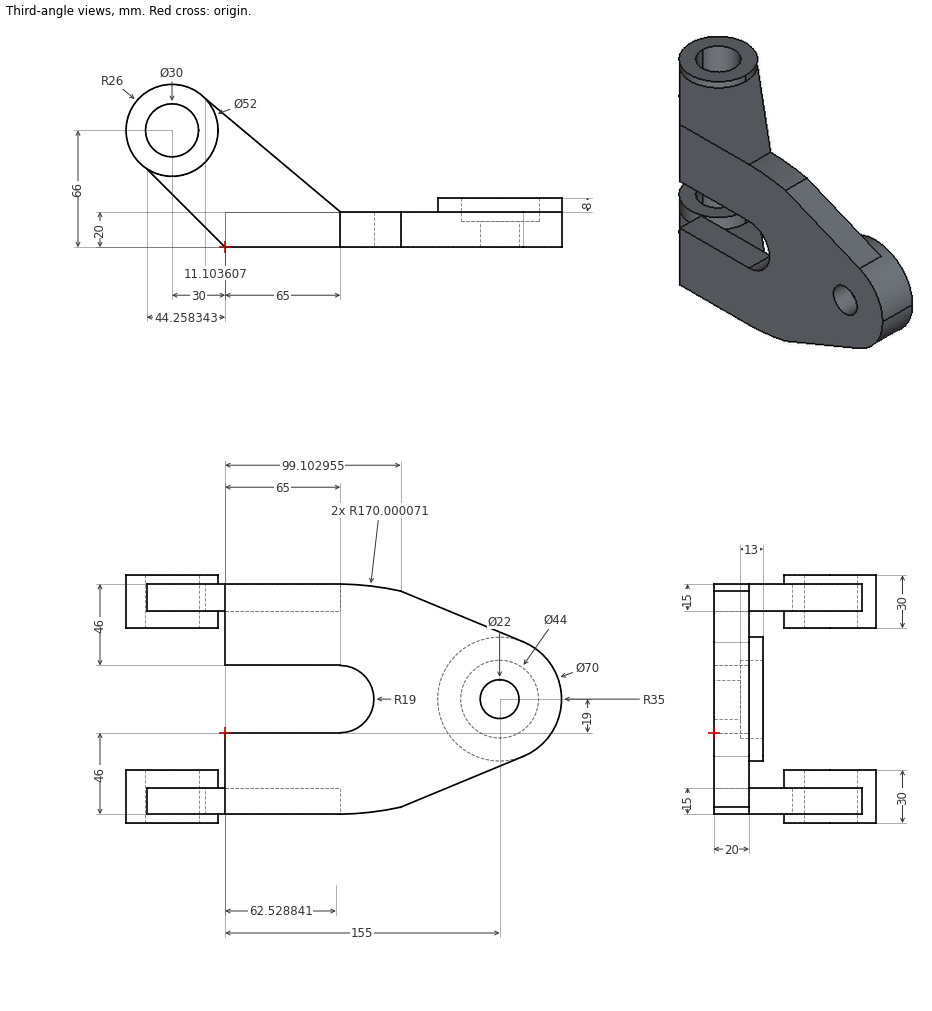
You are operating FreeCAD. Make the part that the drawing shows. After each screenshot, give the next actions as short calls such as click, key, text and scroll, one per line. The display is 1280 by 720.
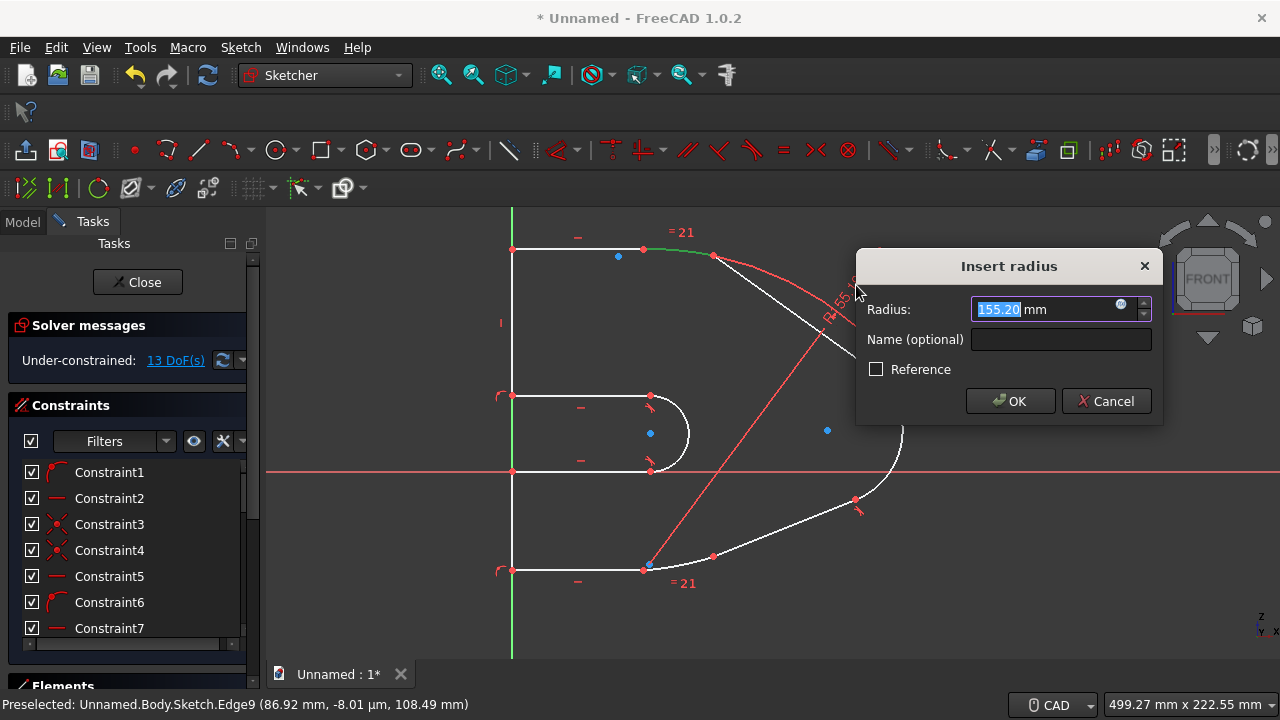
text(170.000071)
key(Return)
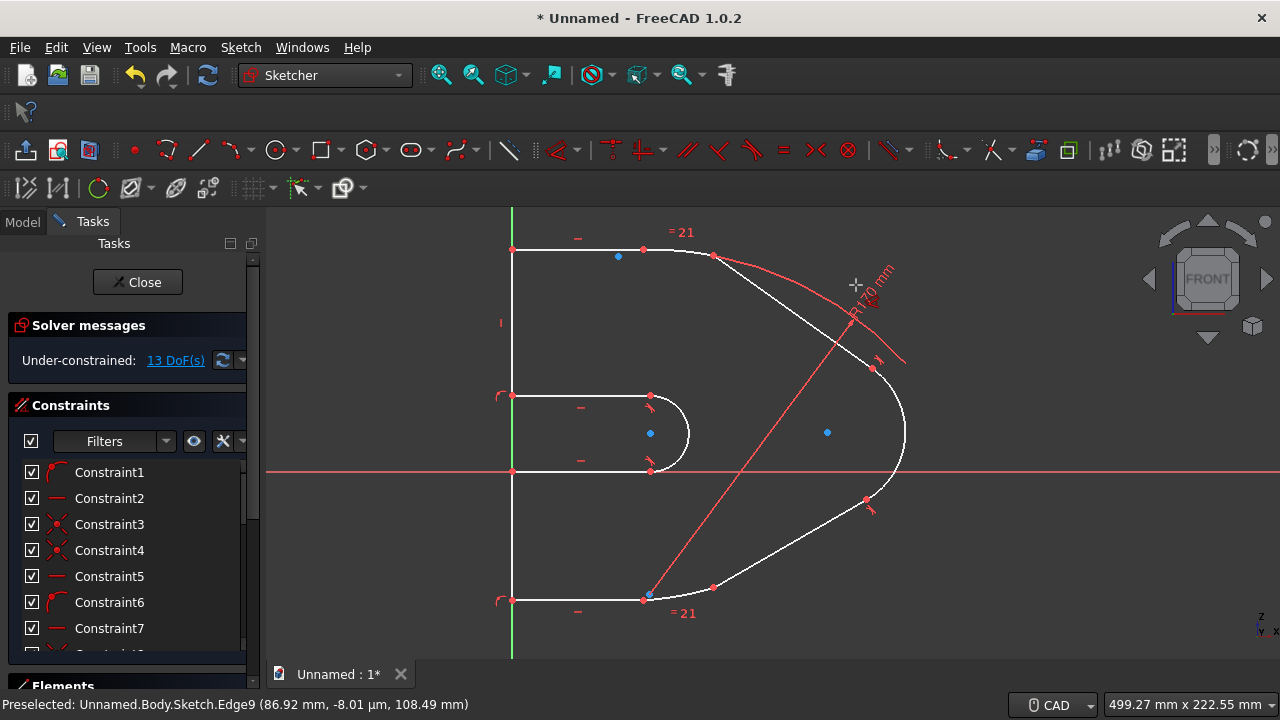
click(901, 406)
click(931, 395)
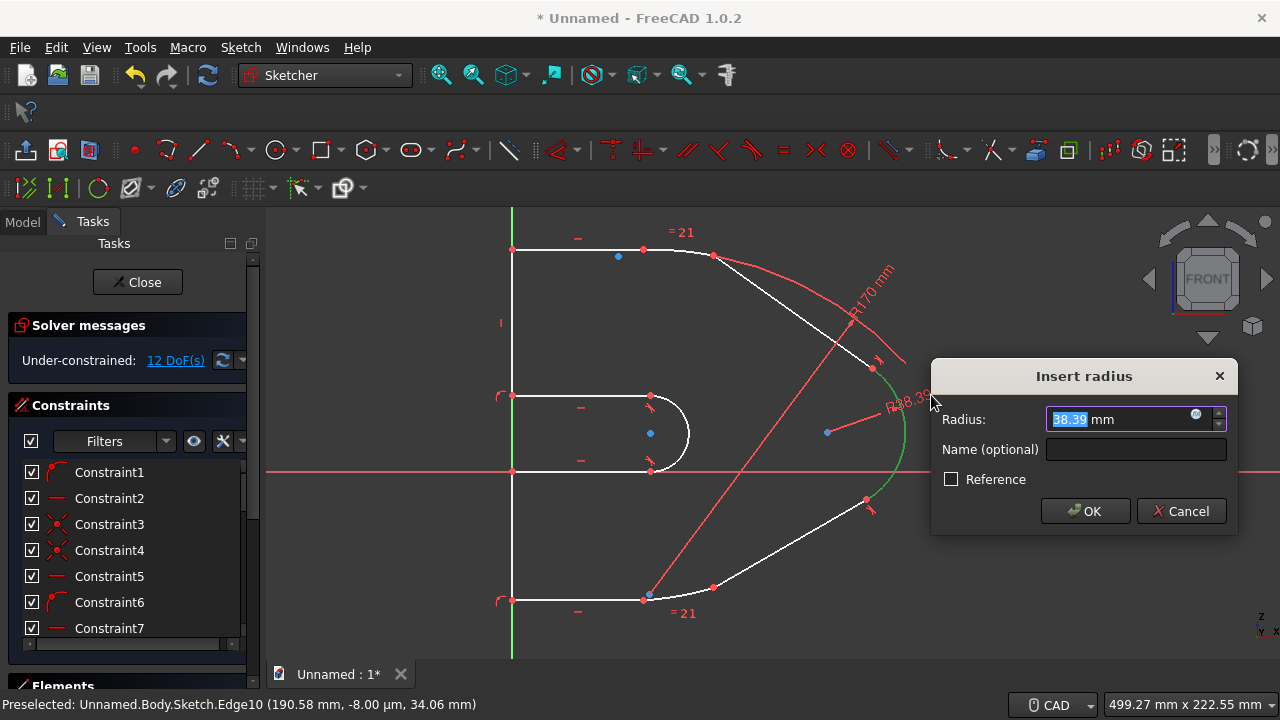
text(35)
key(Return)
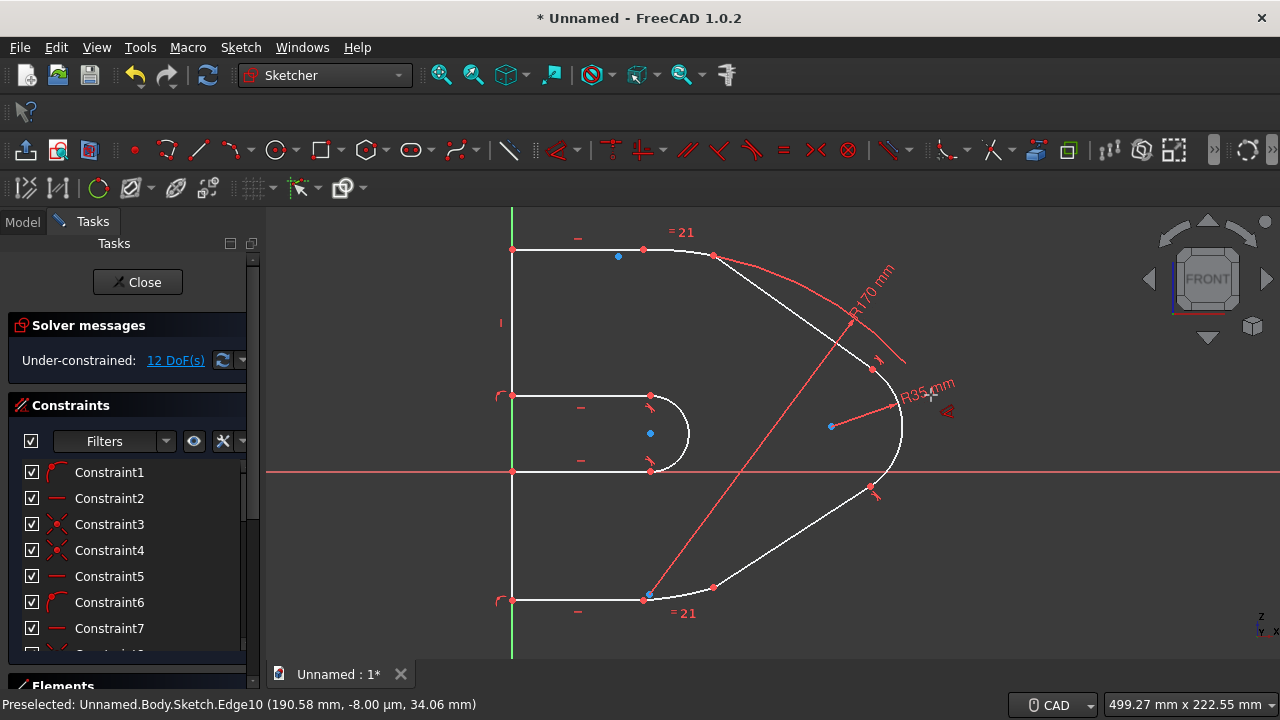
click(682, 456)
click(682, 497)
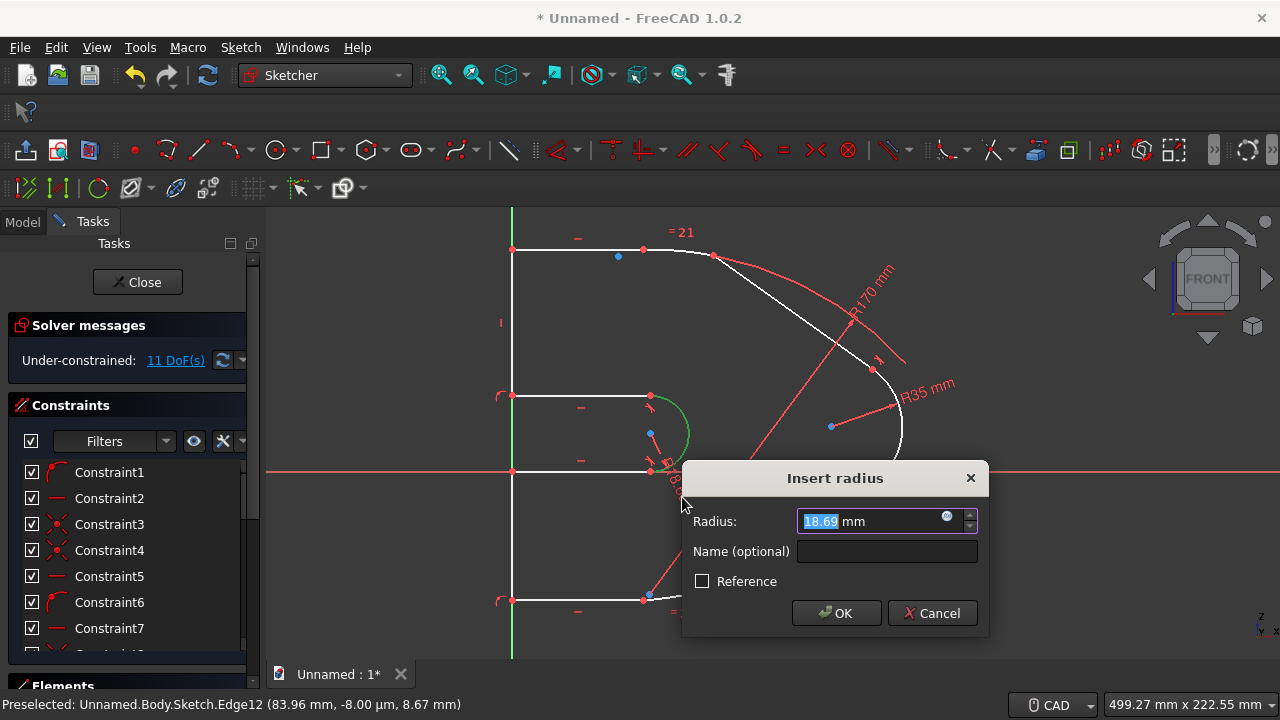
text(19)
key(Return)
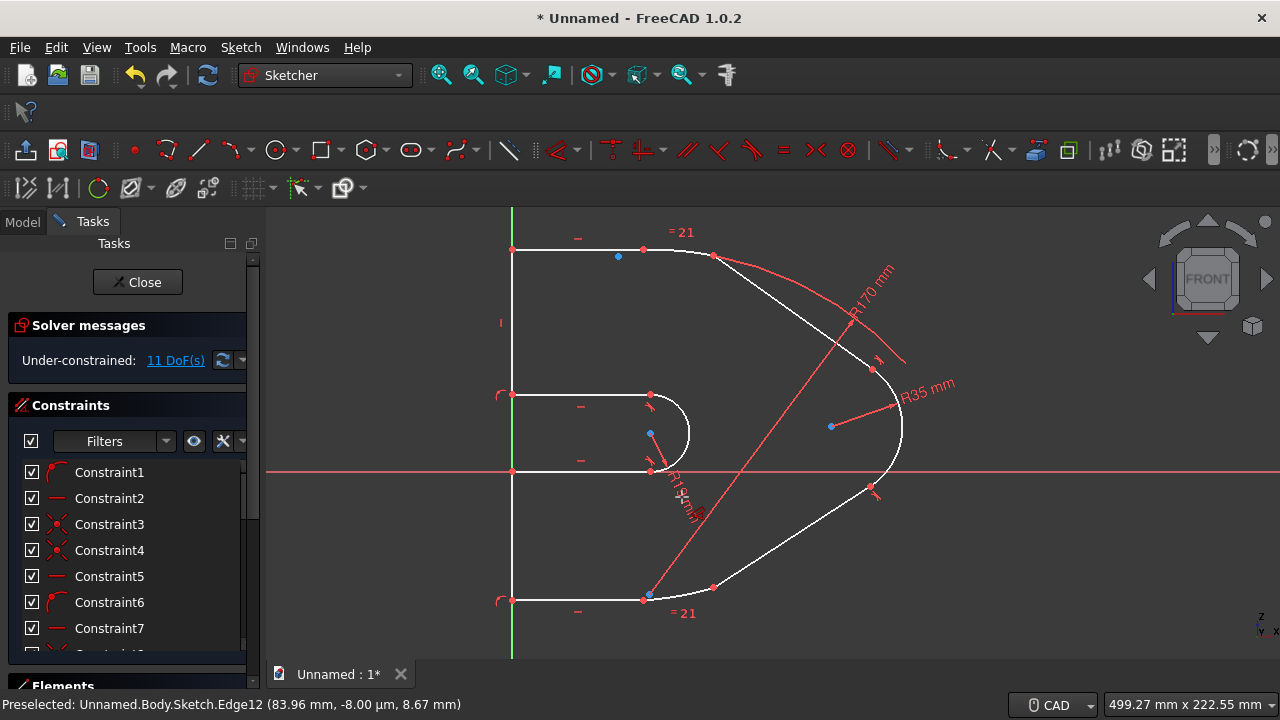
click(609, 395)
click(582, 361)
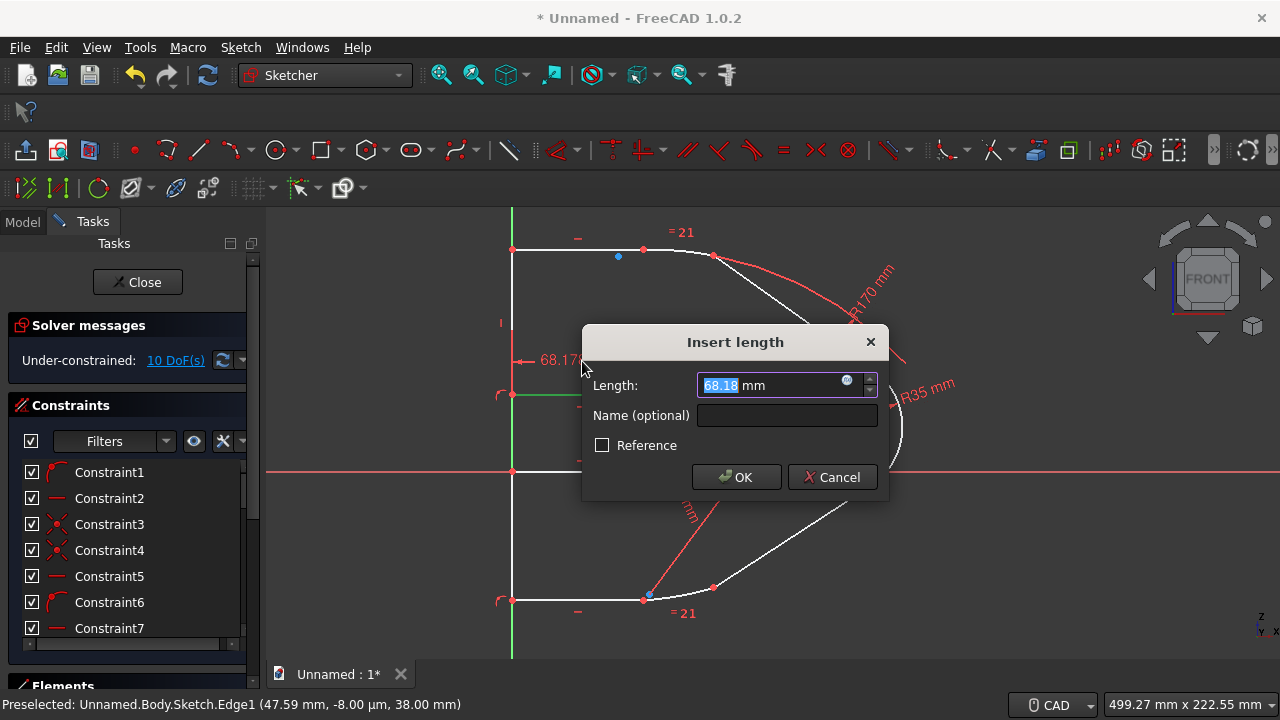
text(65)
key(Return)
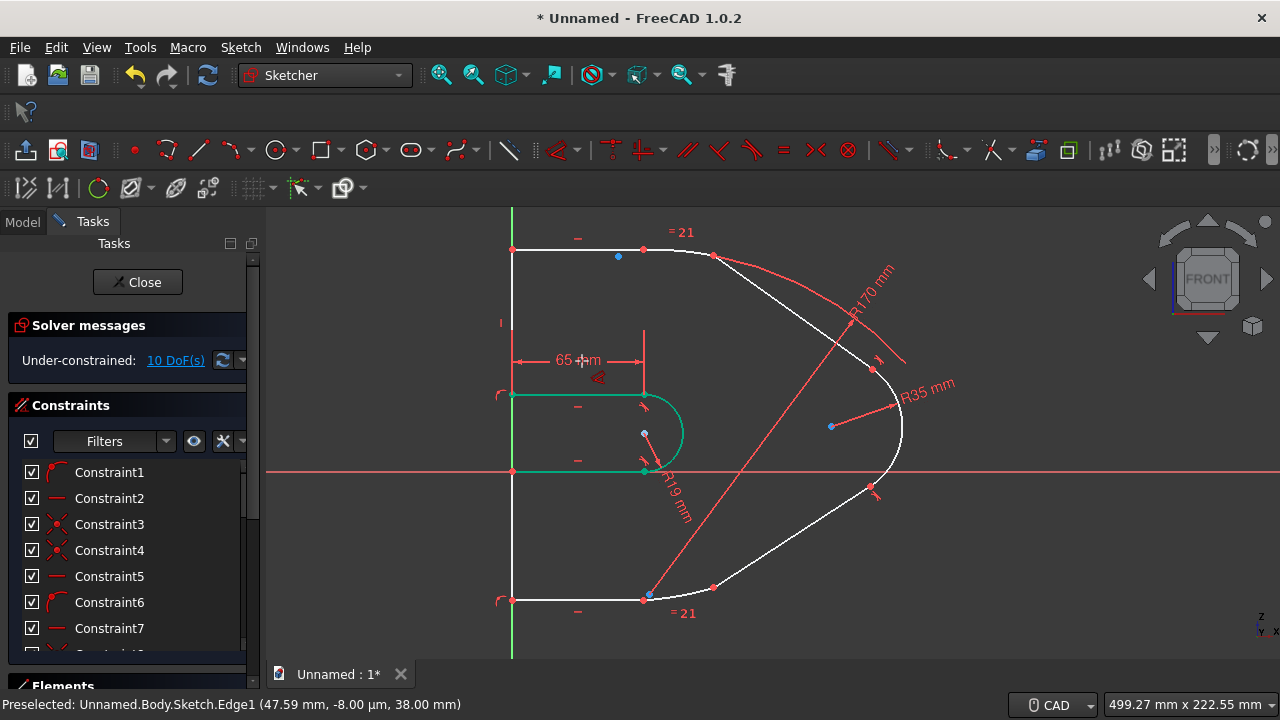
click(512, 351)
click(478, 322)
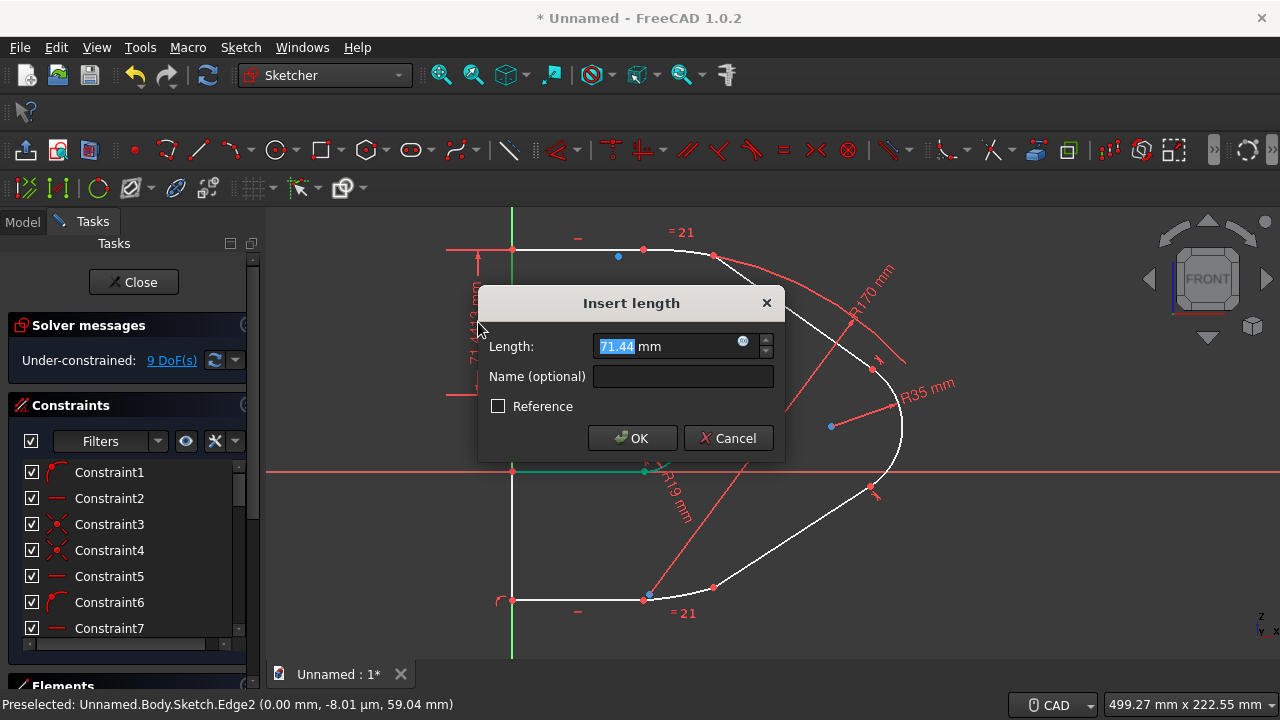
text(46)
key(Return)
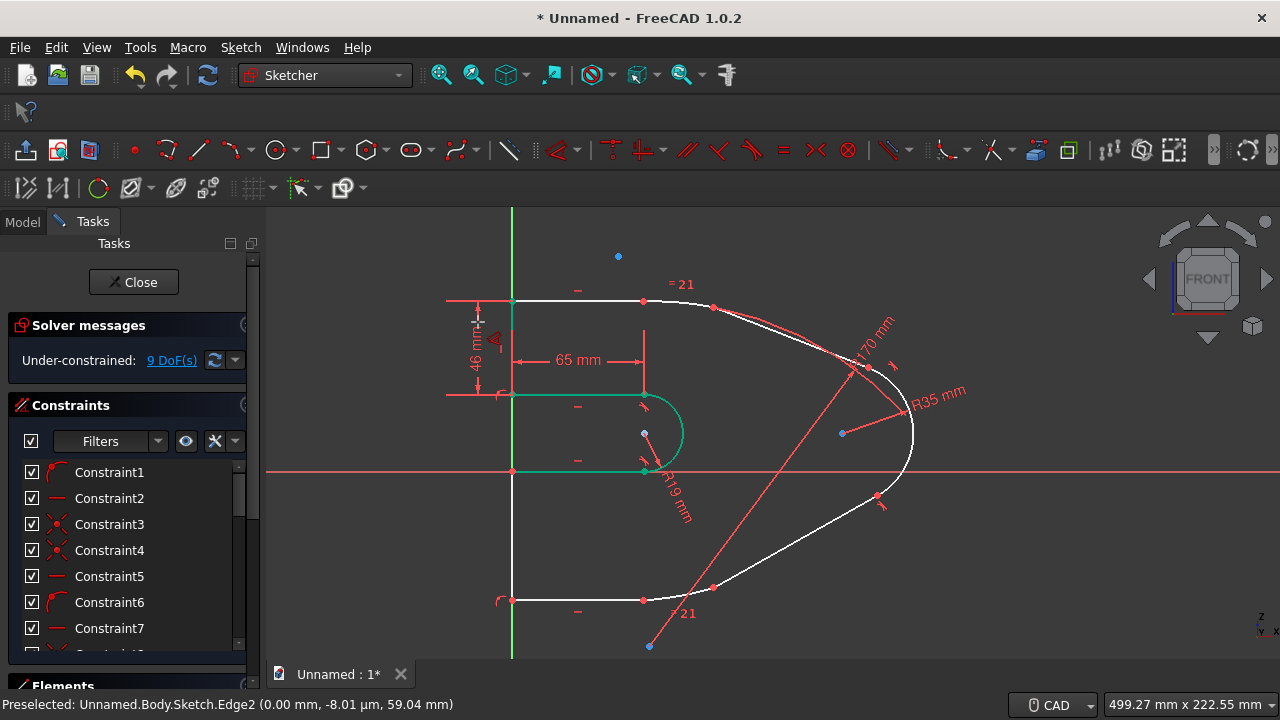
click(552, 301)
click(578, 267)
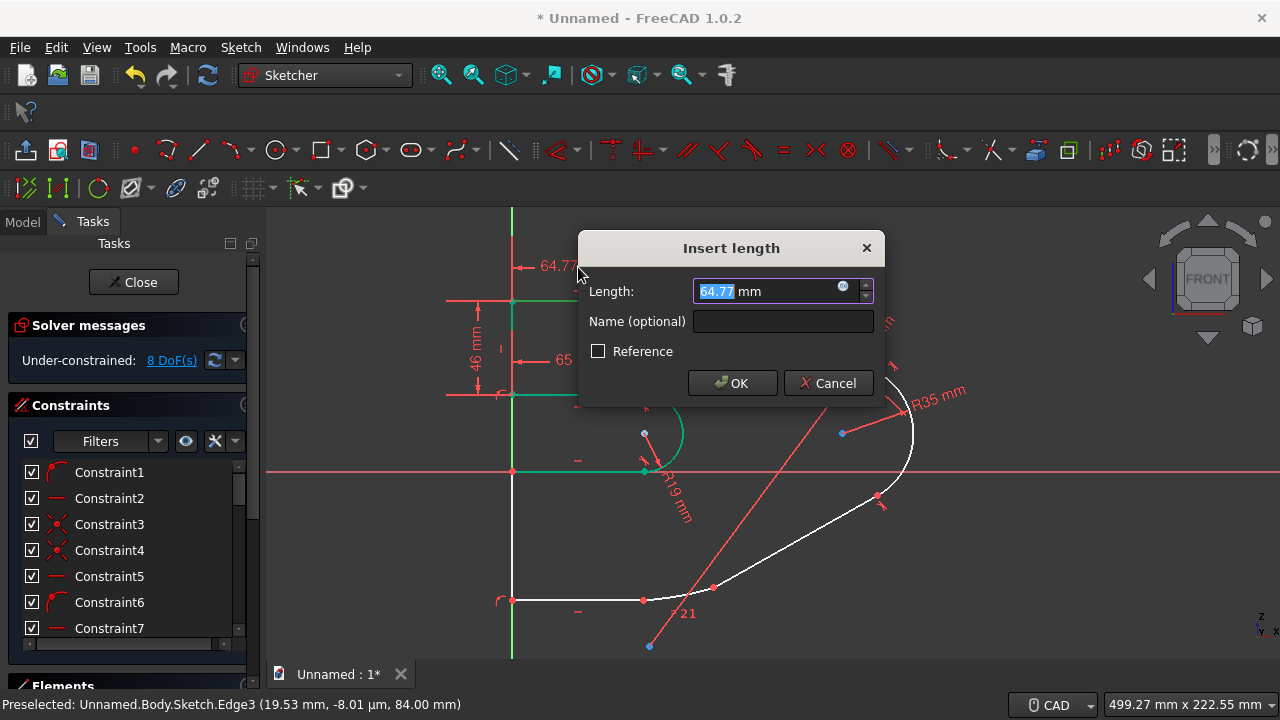
text(65)
key(Return)